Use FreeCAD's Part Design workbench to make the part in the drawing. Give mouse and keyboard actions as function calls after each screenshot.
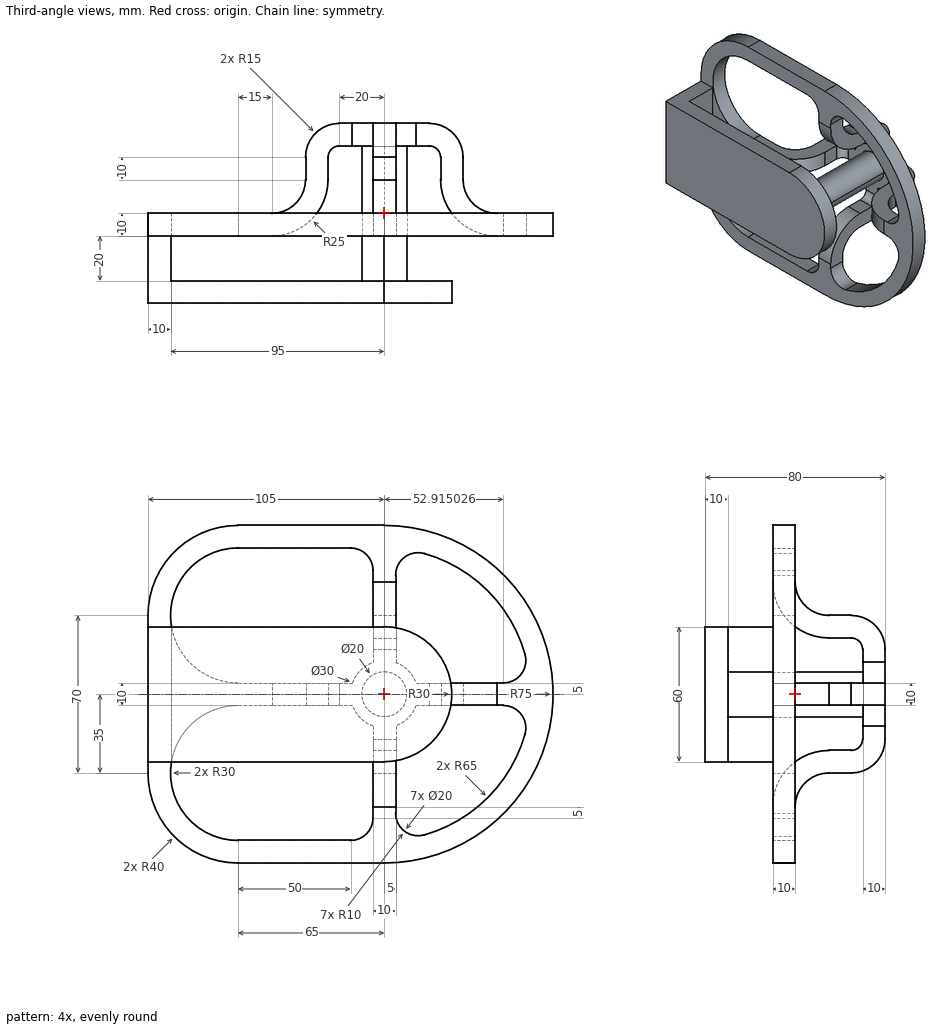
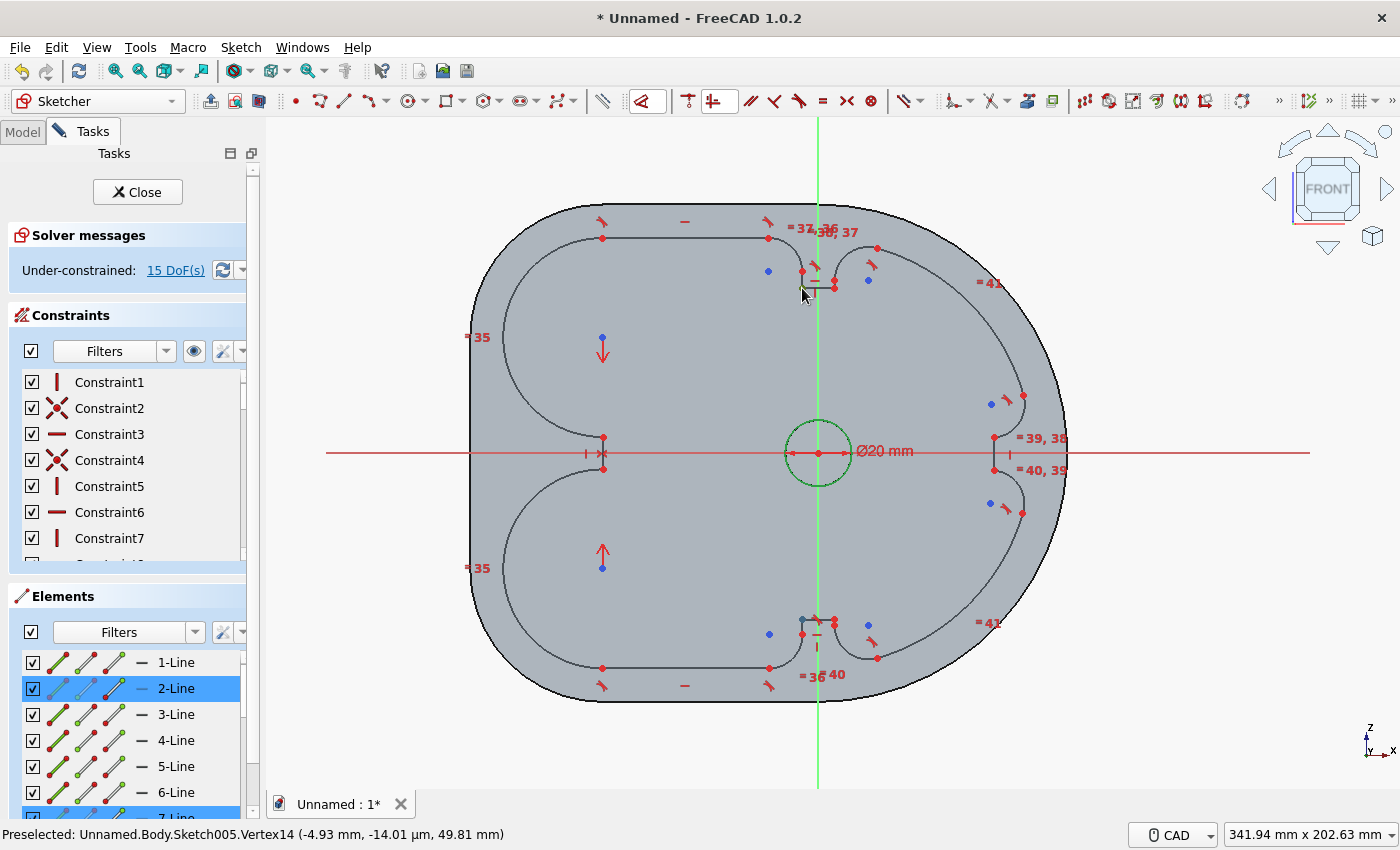
click(361, 453)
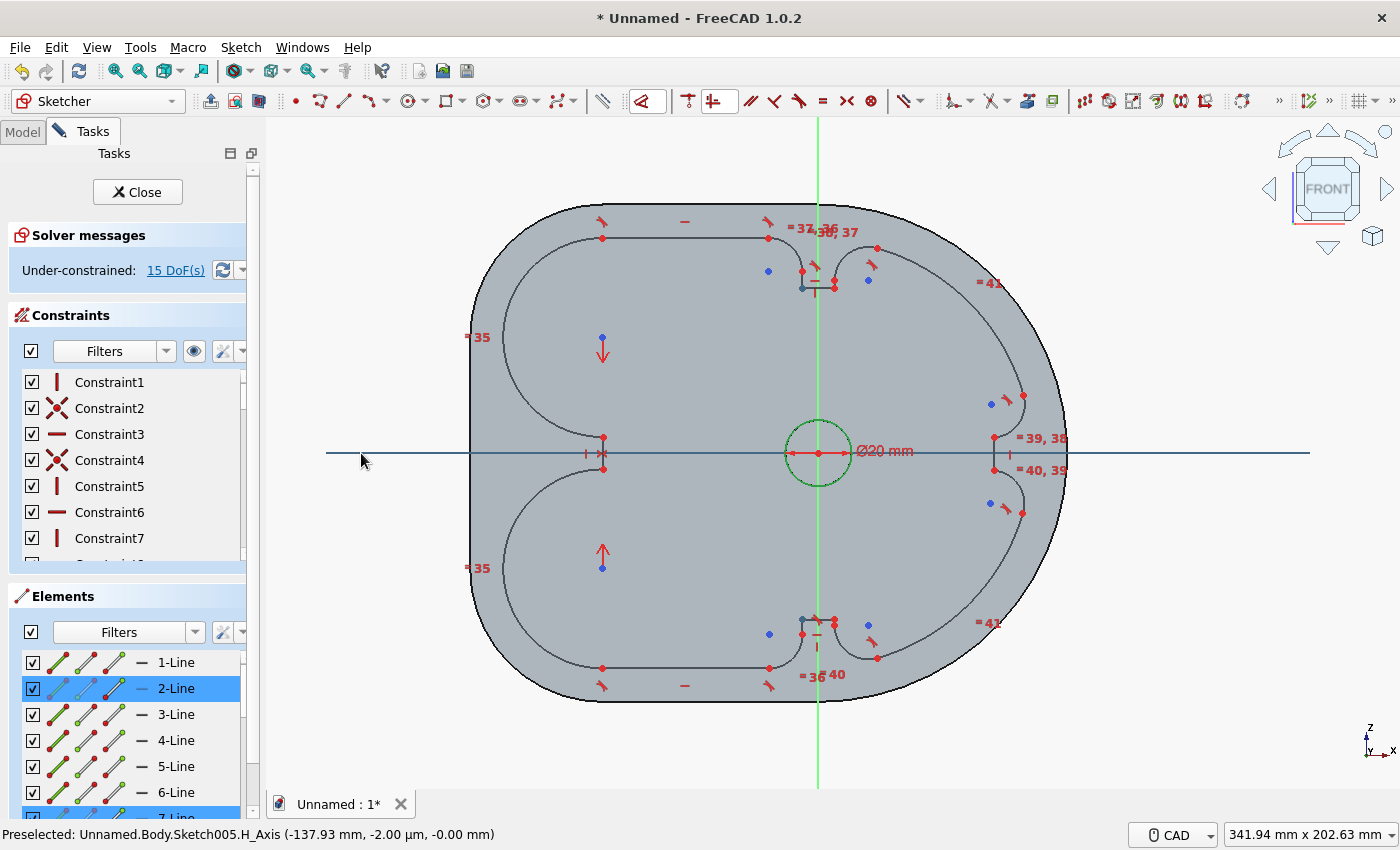
click(848, 102)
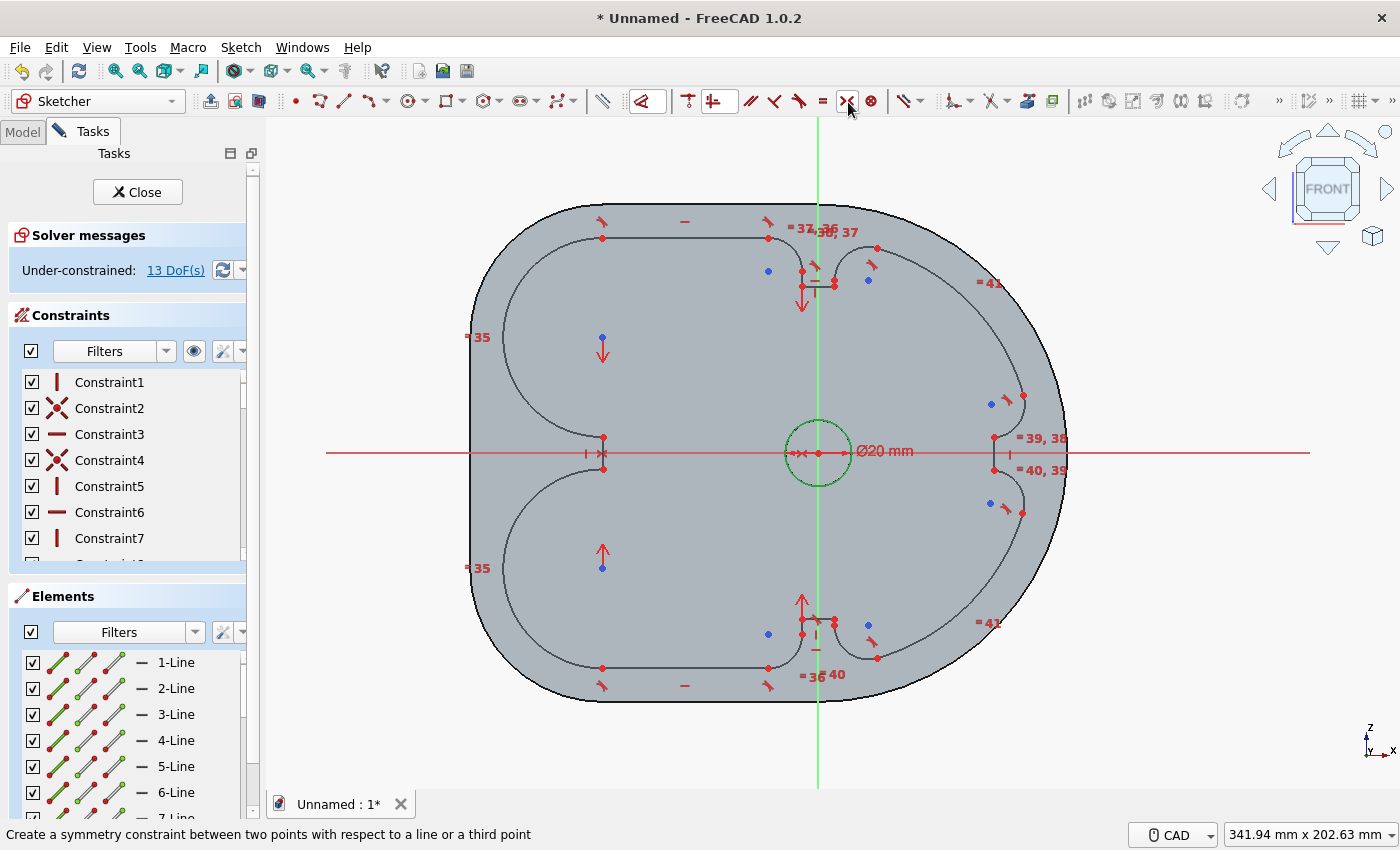
click(784, 665)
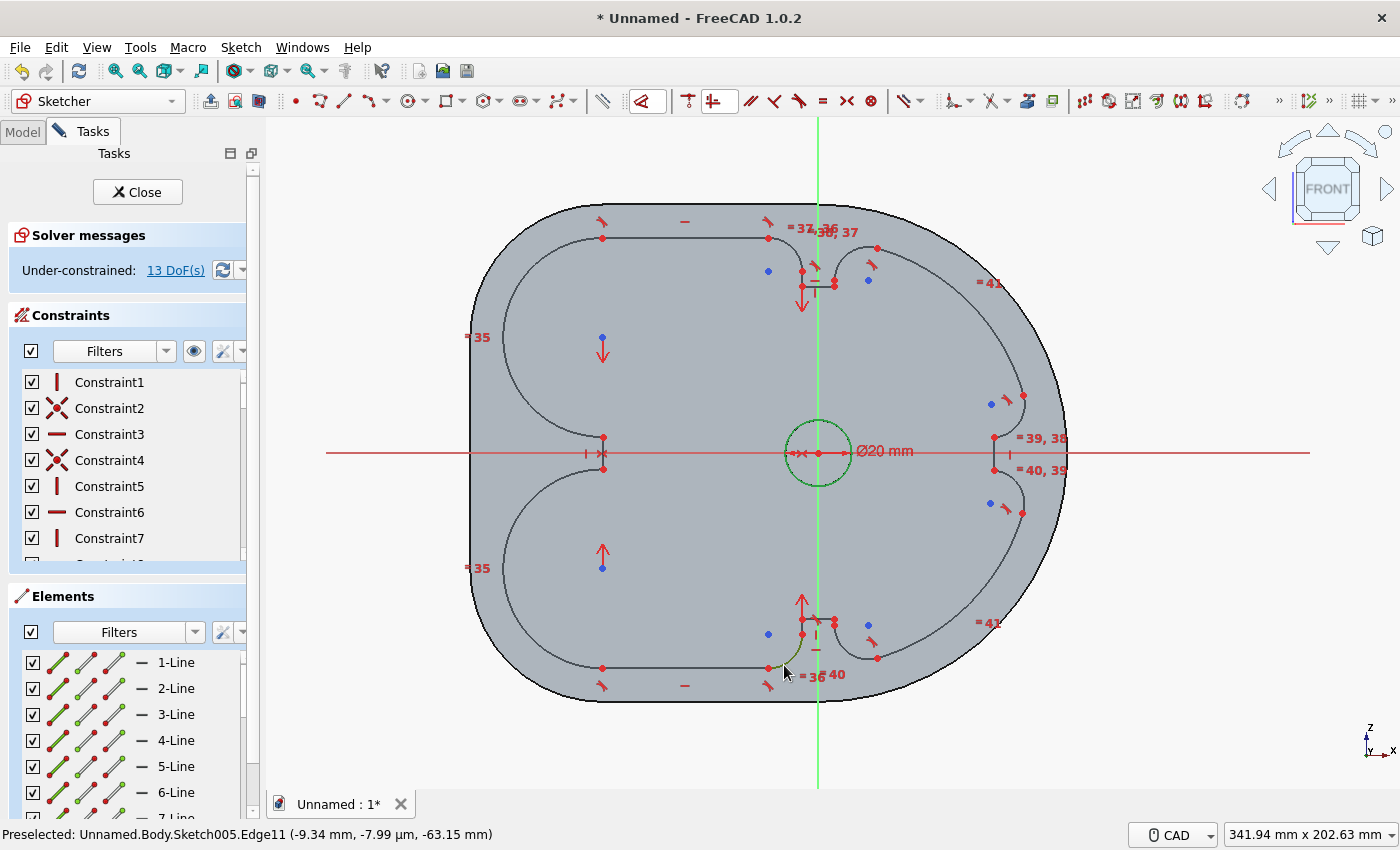
key(k)
key(r)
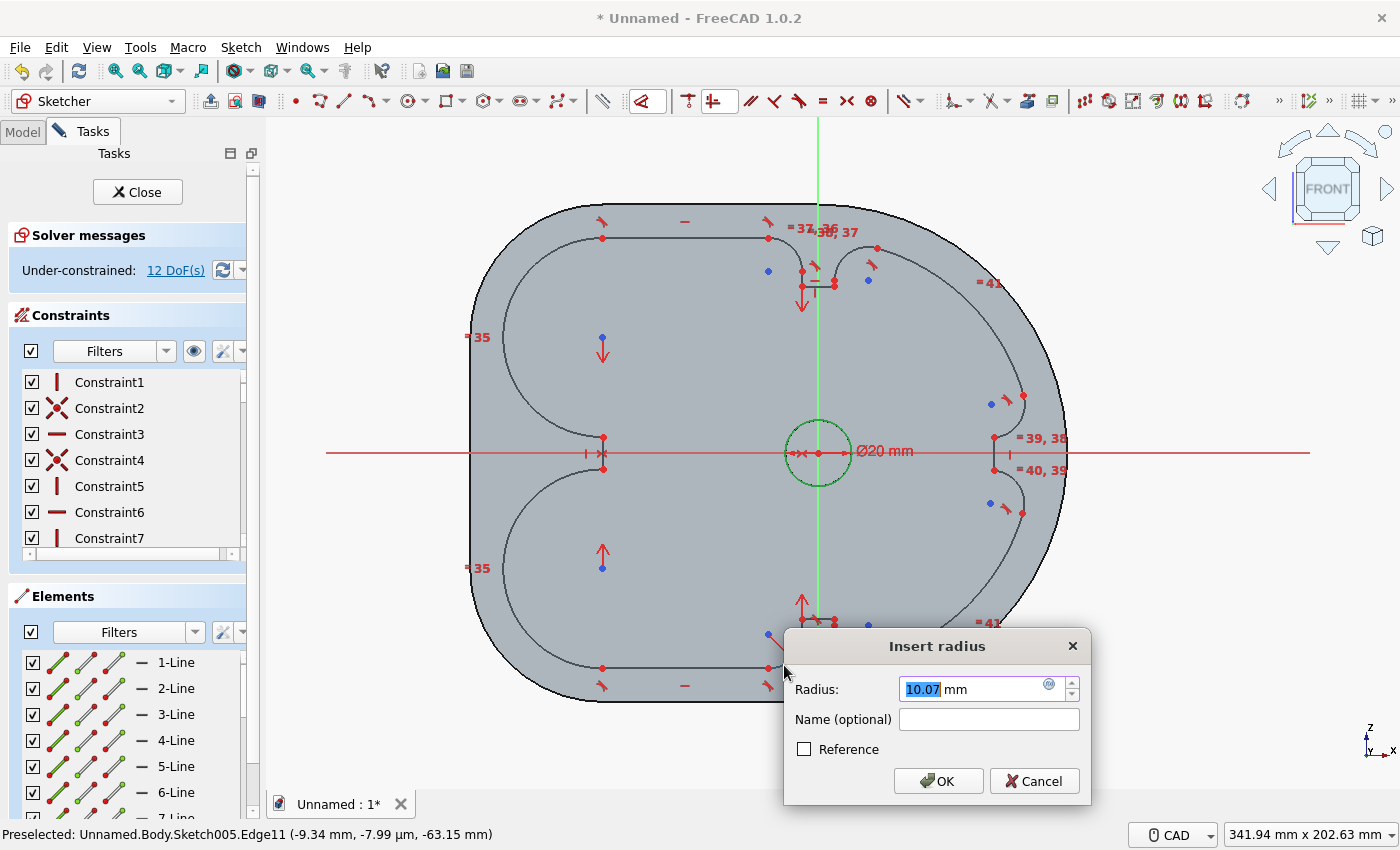
text(10)
key(Return)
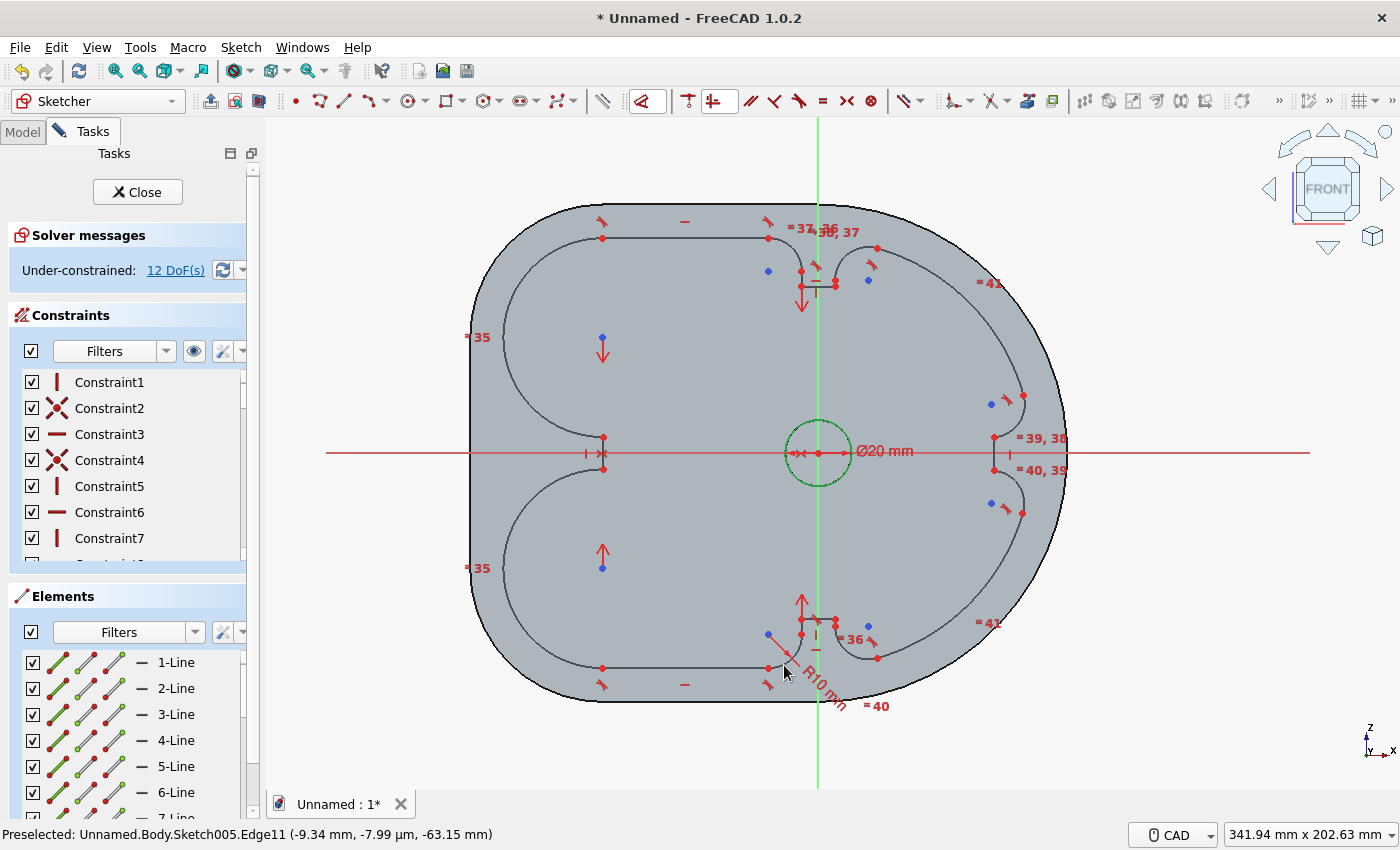
click(522, 510)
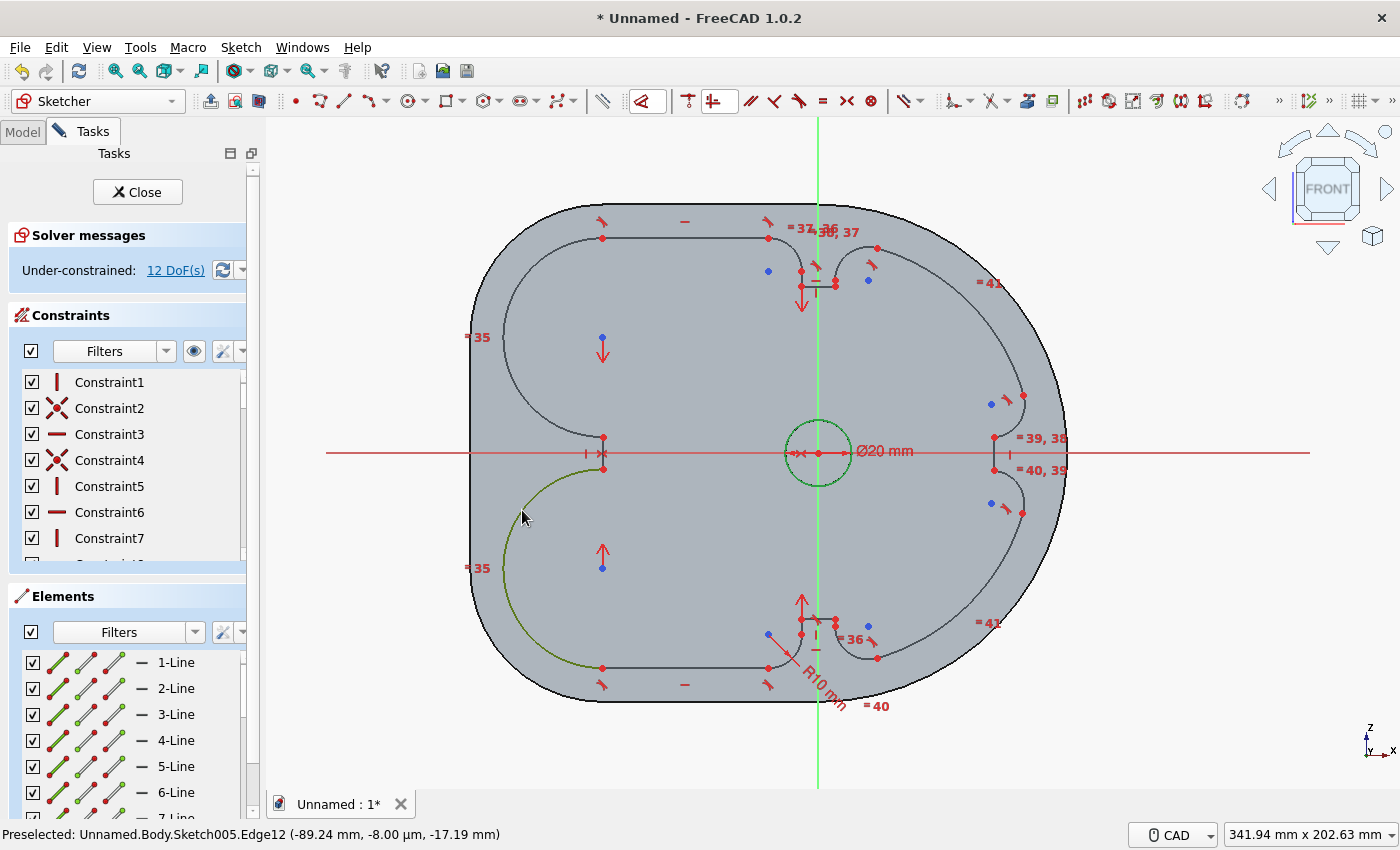
click(660, 102)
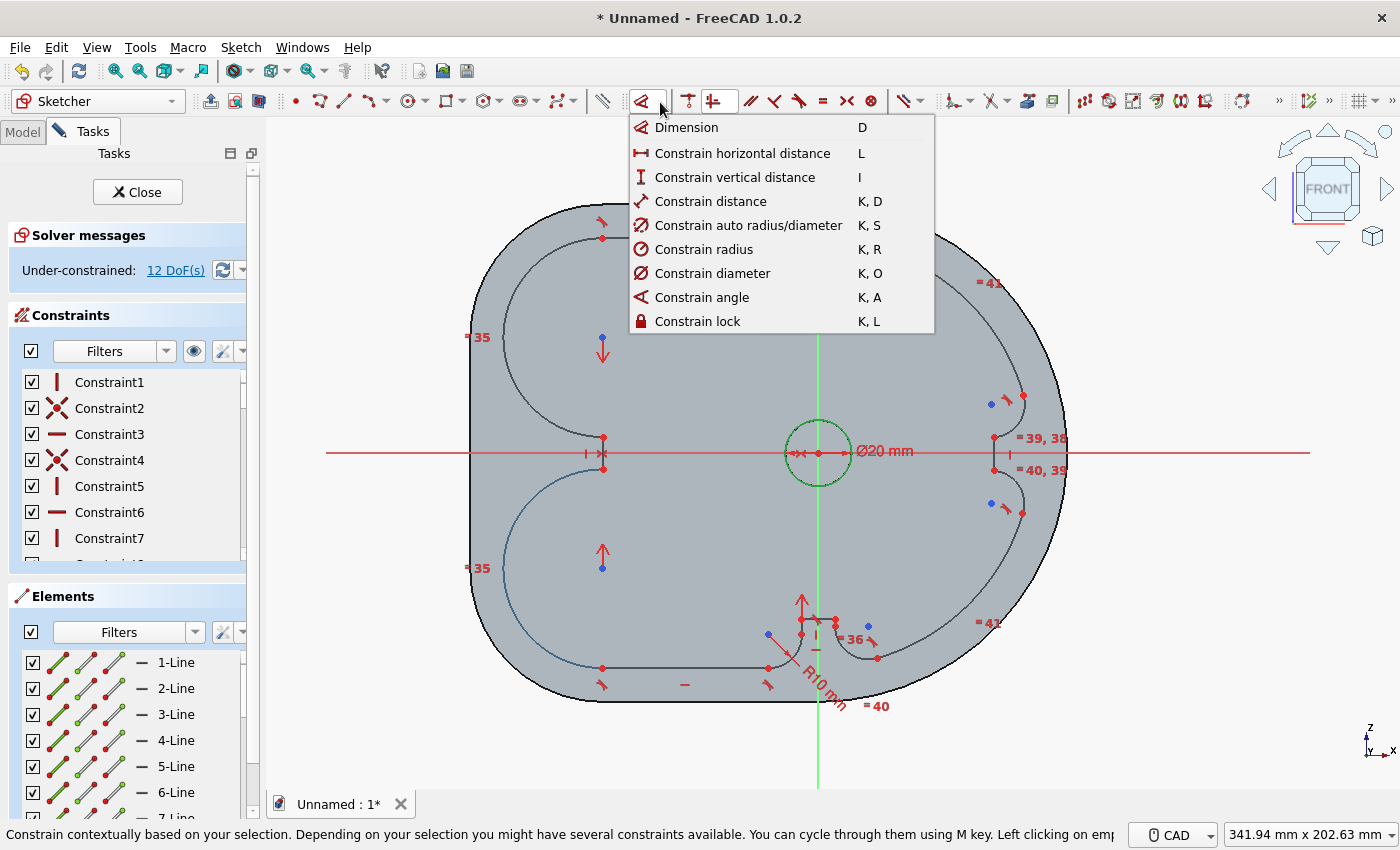
click(782, 249)